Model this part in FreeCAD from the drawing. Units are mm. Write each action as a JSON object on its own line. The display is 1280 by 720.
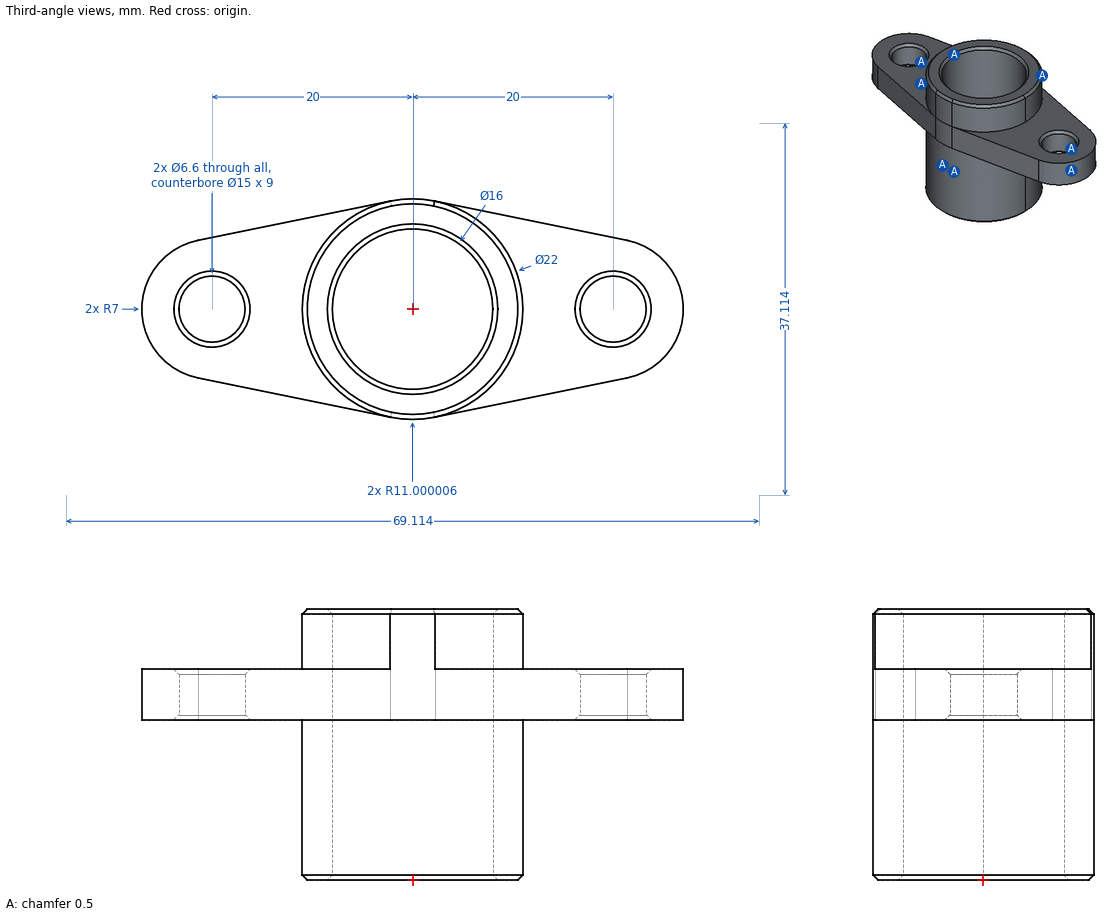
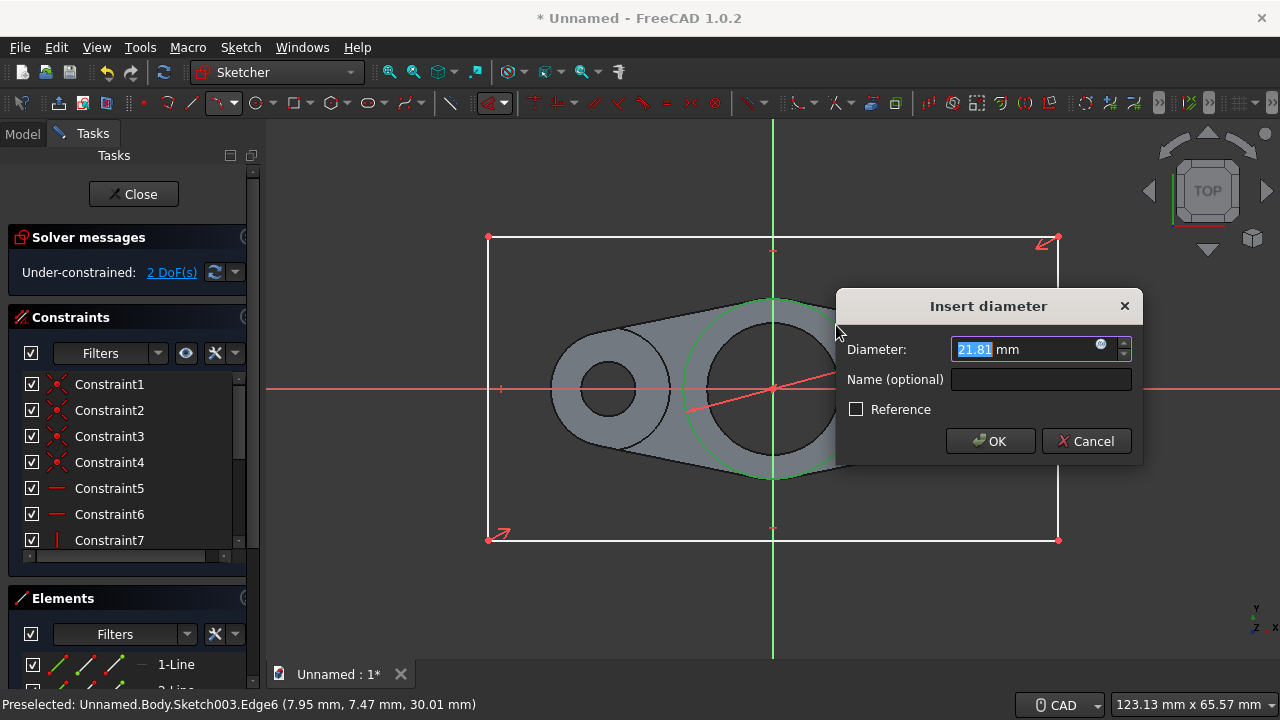
{"action": "type", "text": "22"}
{"action": "key", "text": "Return"}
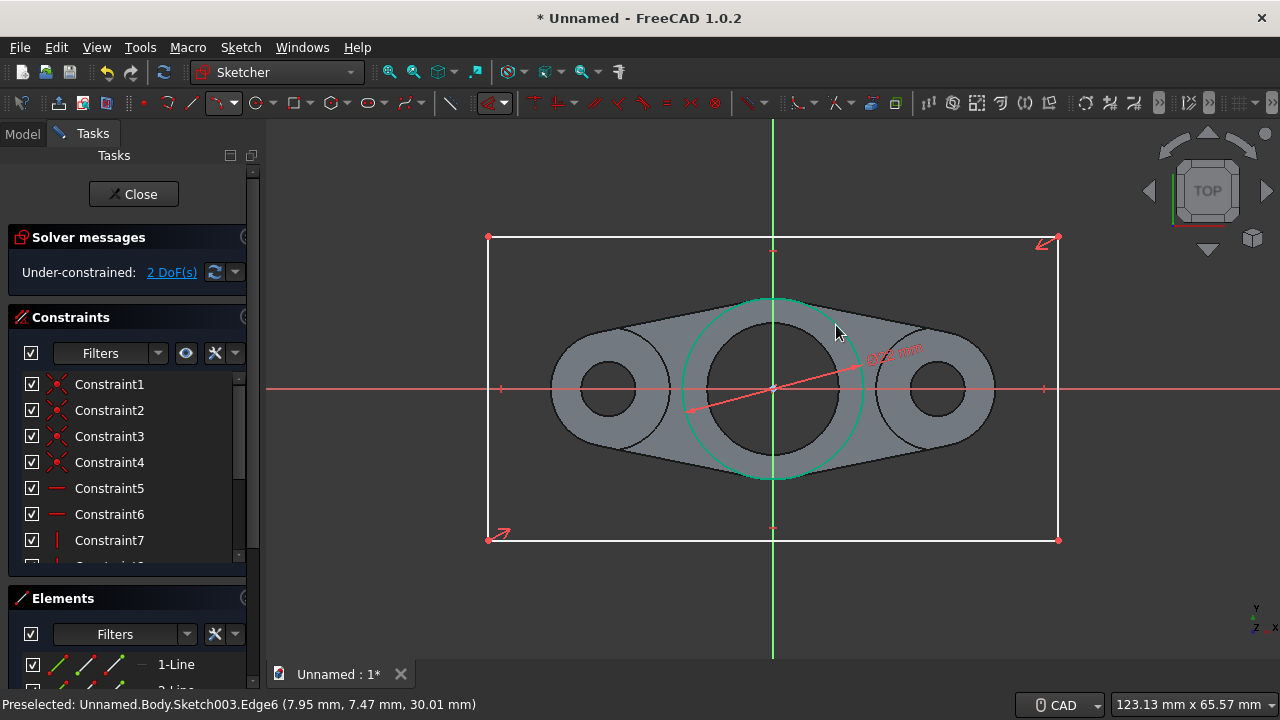
{"action": "left_click", "coordinate": [659, 541]}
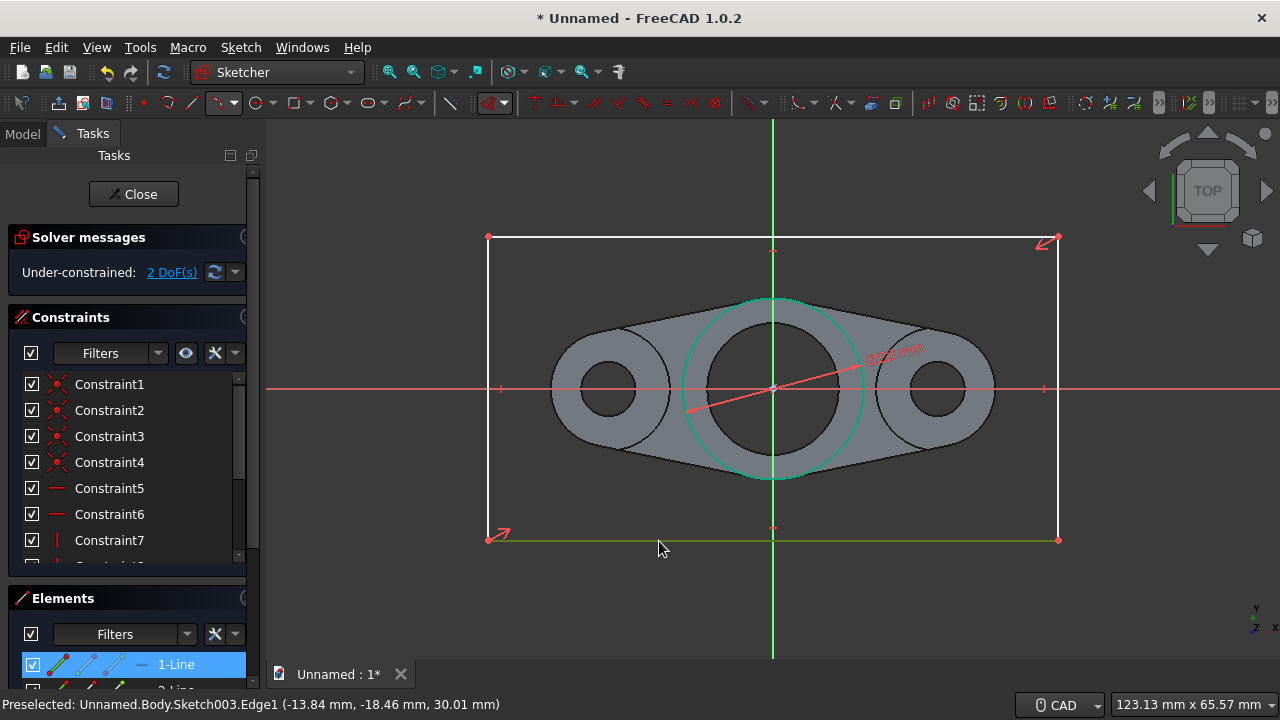
{"action": "left_click", "coordinate": [506, 104]}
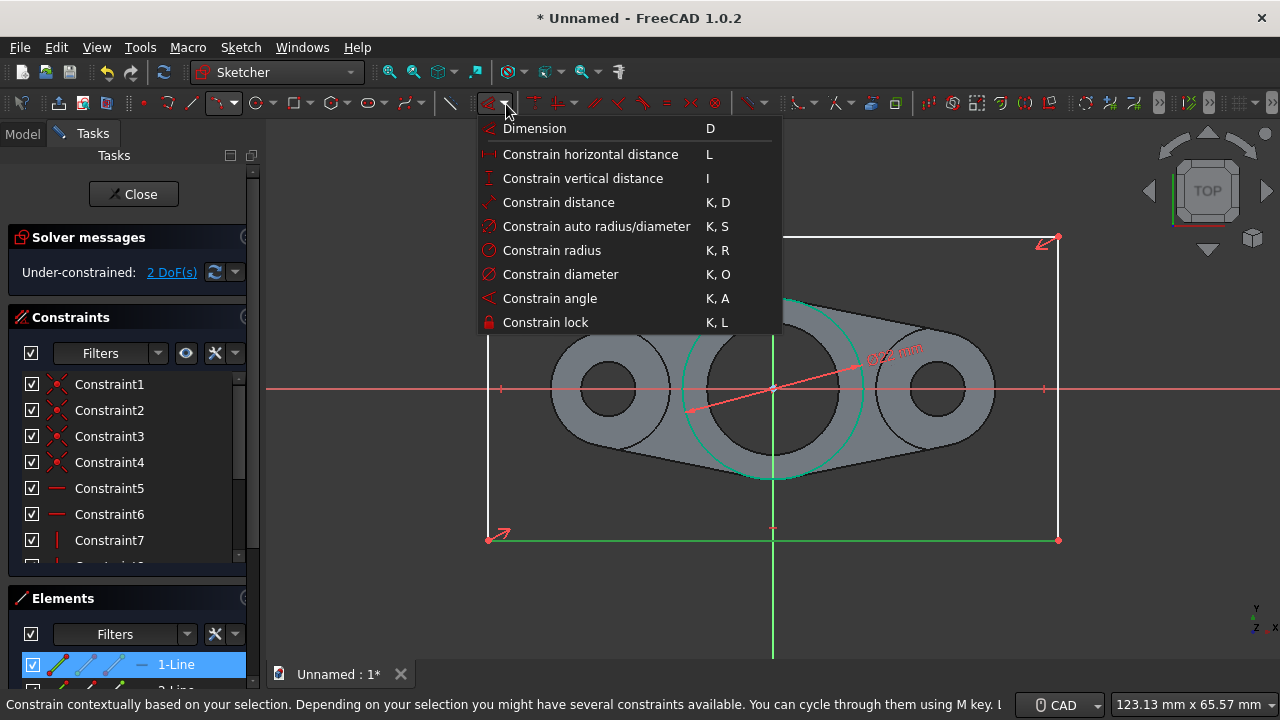
{"action": "left_click", "coordinate": [630, 154]}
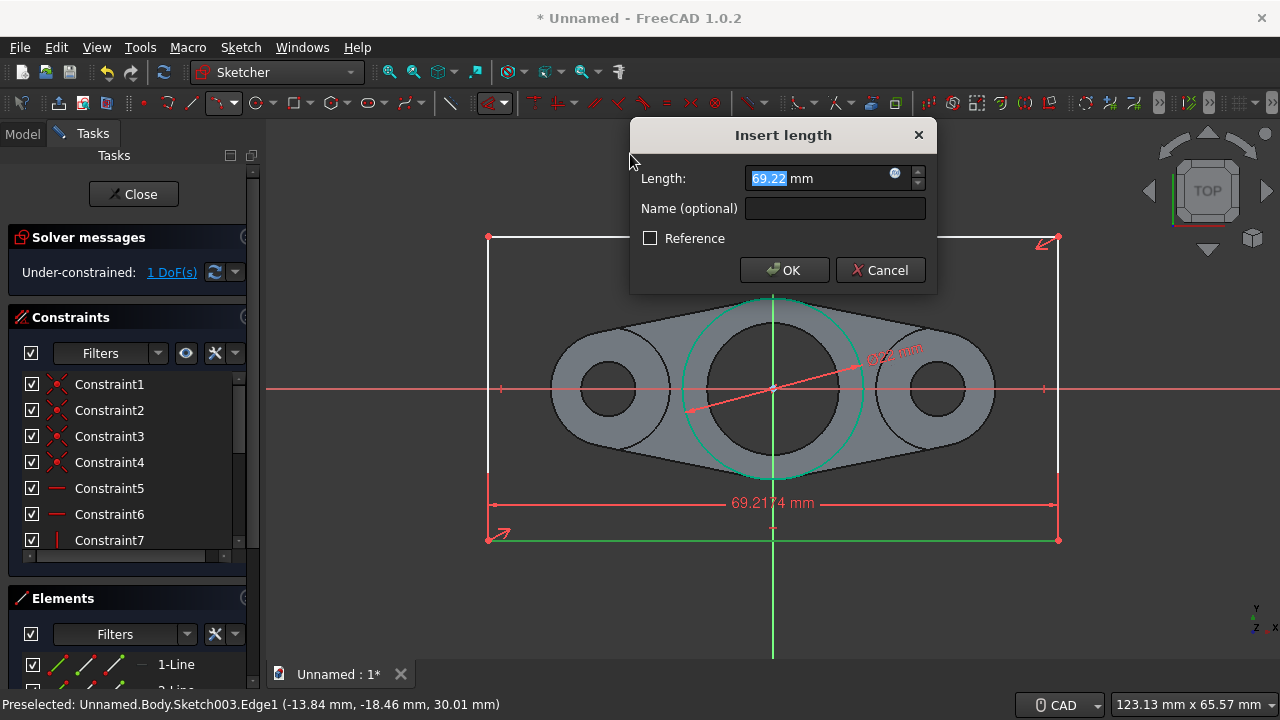
{"action": "type", "text": "69.114"}
{"action": "key", "text": "Return"}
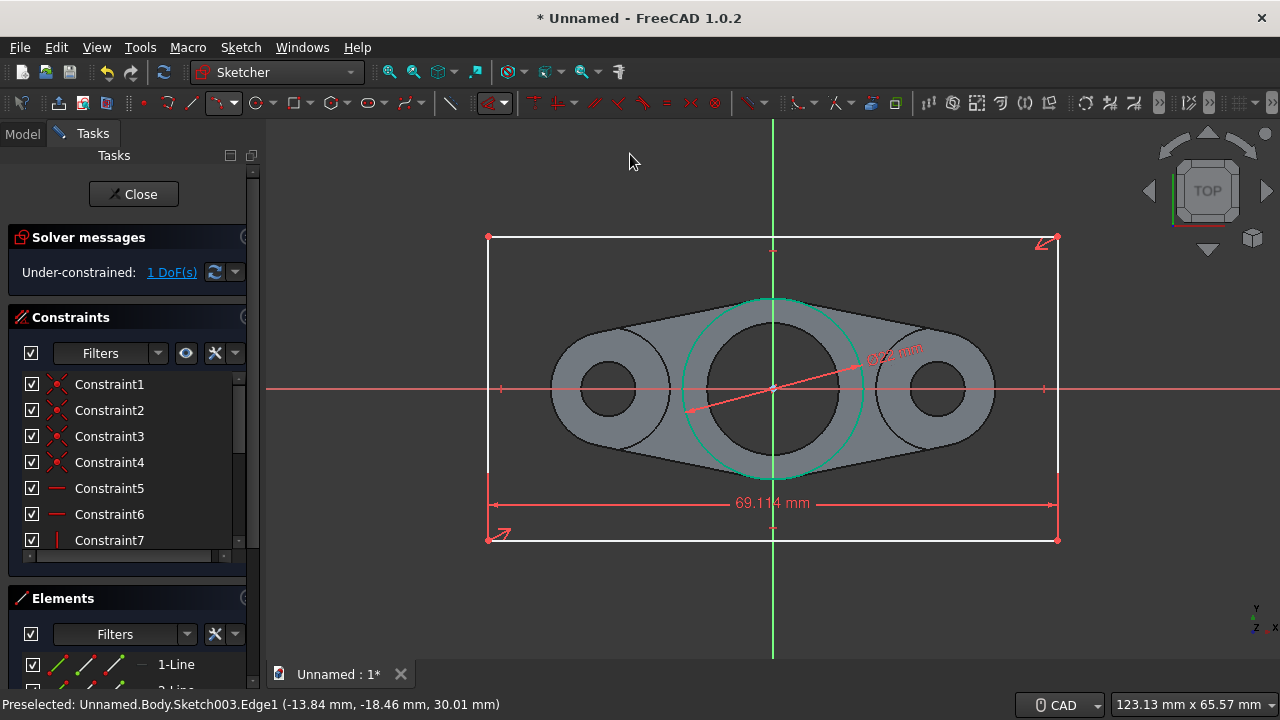
{"action": "left_click", "coordinate": [1058, 450]}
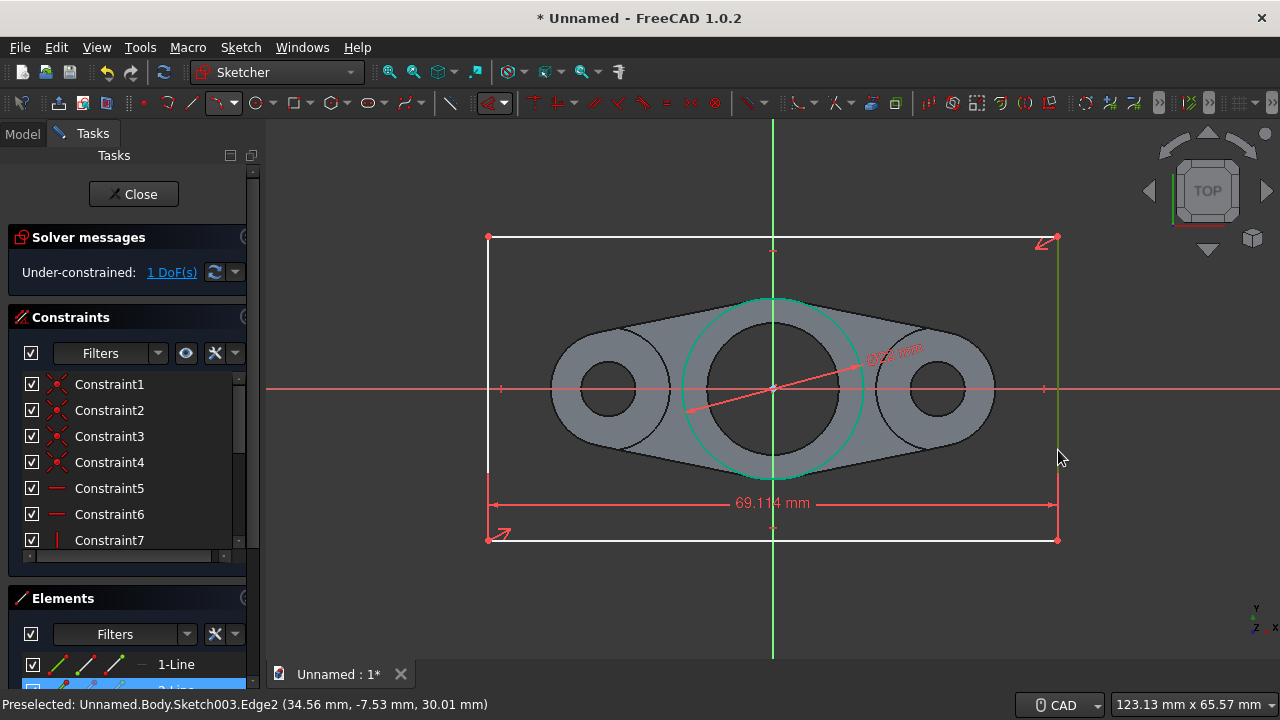
{"action": "key", "text": "i"}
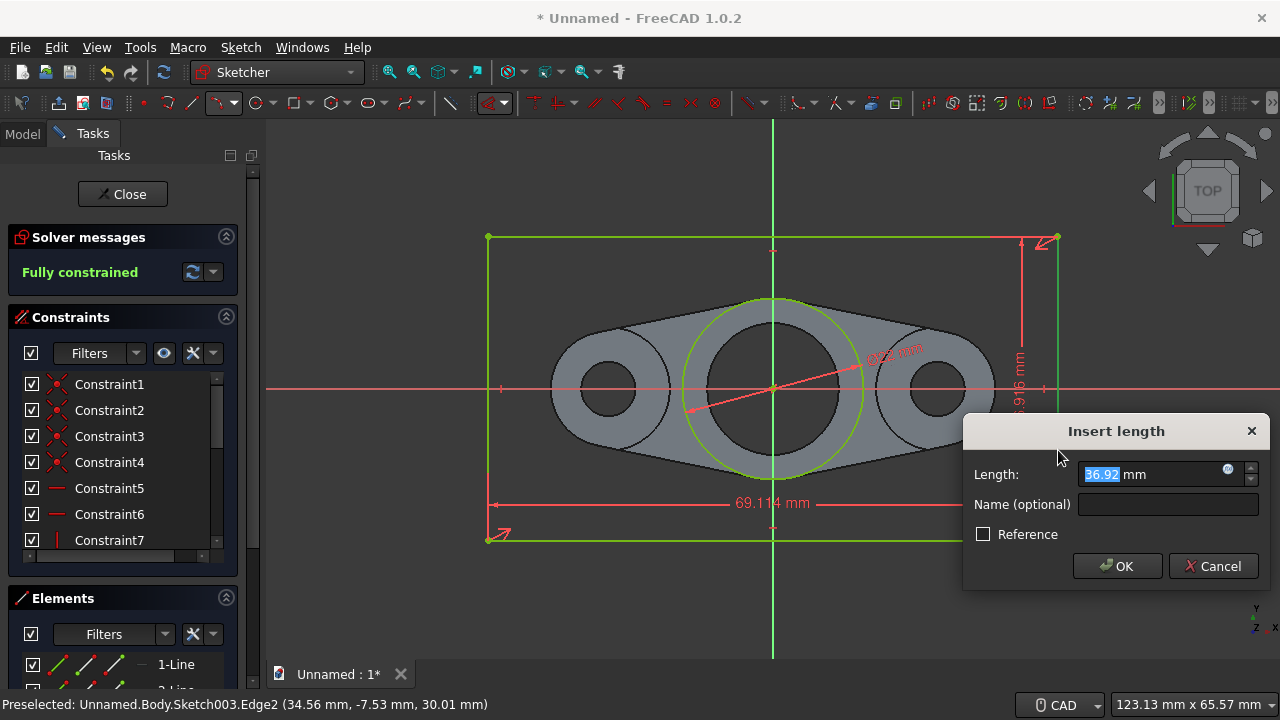
{"action": "type", "text": "37.114"}
{"action": "key", "text": "Return"}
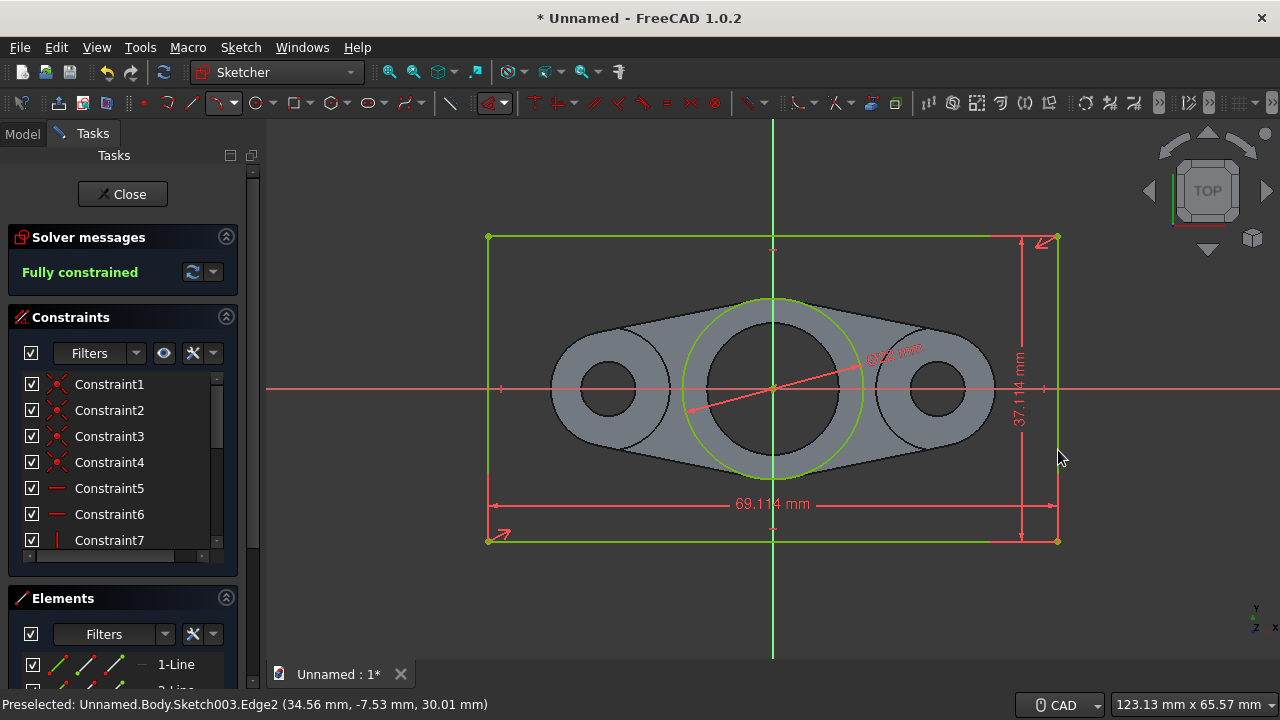
{"action": "left_click", "coordinate": [123, 194]}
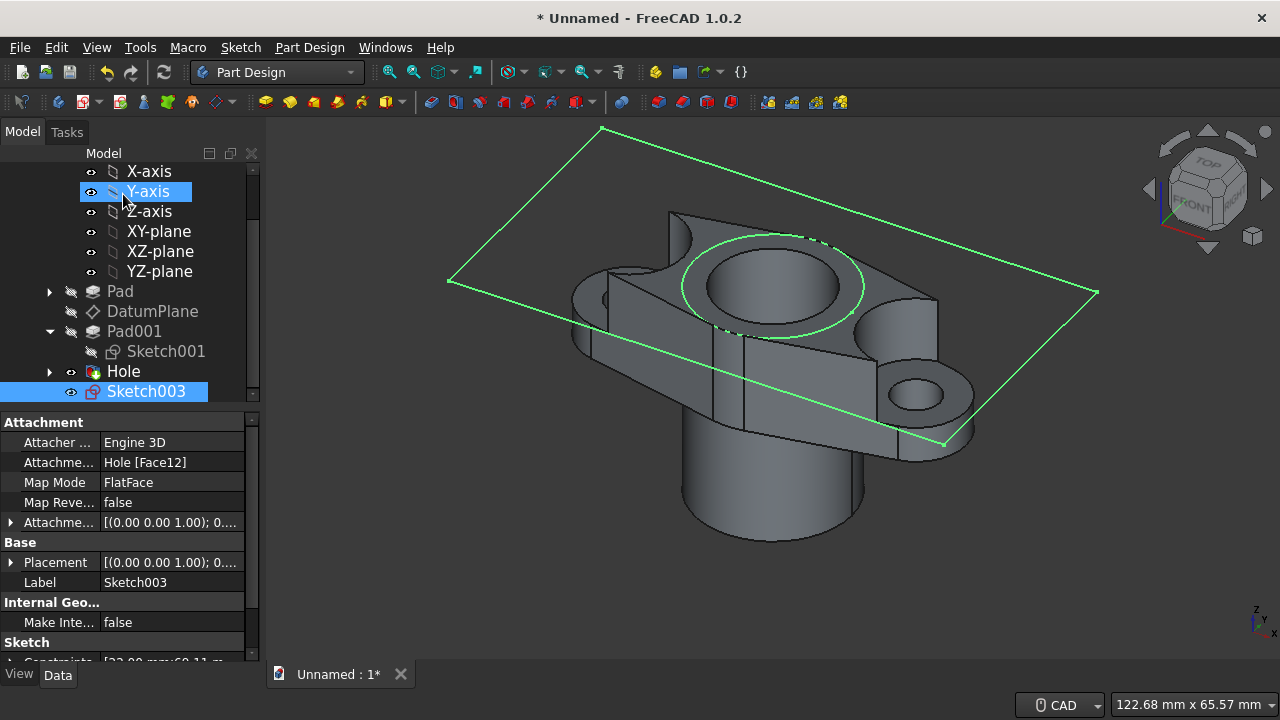
{"action": "left_click", "coordinate": [432, 102]}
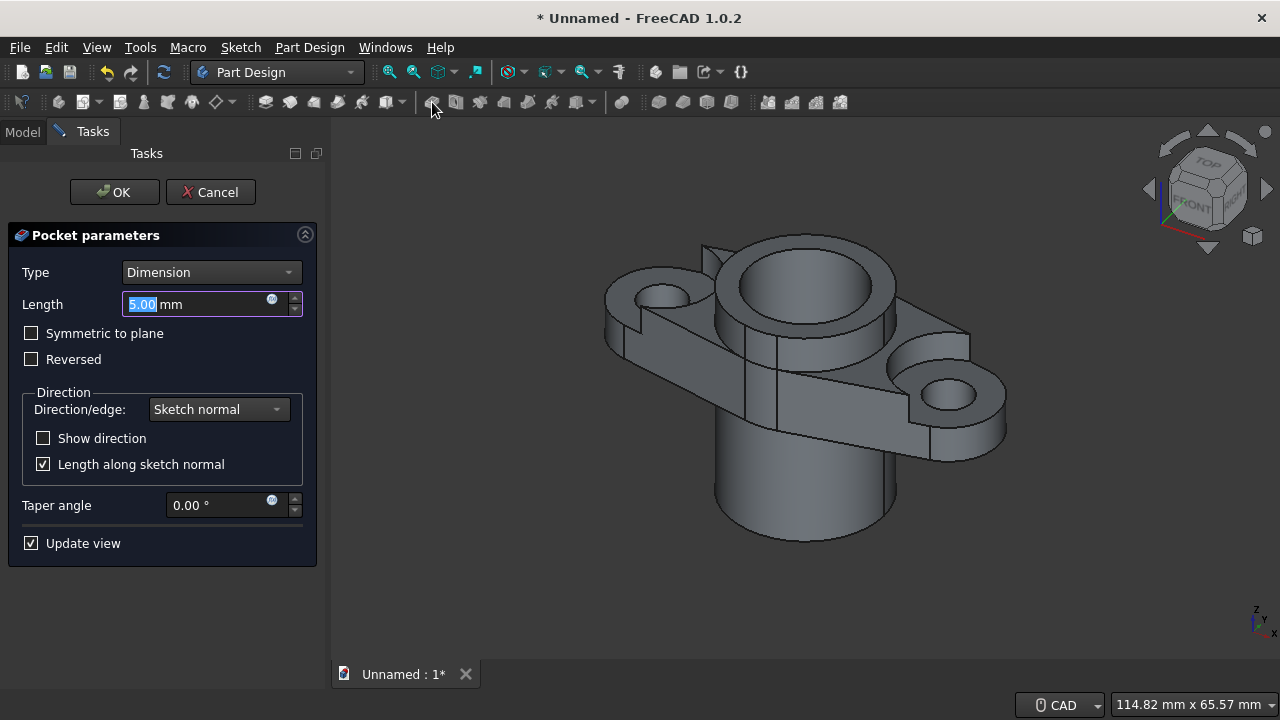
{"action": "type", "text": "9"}
{"action": "key", "text": "Tab"}